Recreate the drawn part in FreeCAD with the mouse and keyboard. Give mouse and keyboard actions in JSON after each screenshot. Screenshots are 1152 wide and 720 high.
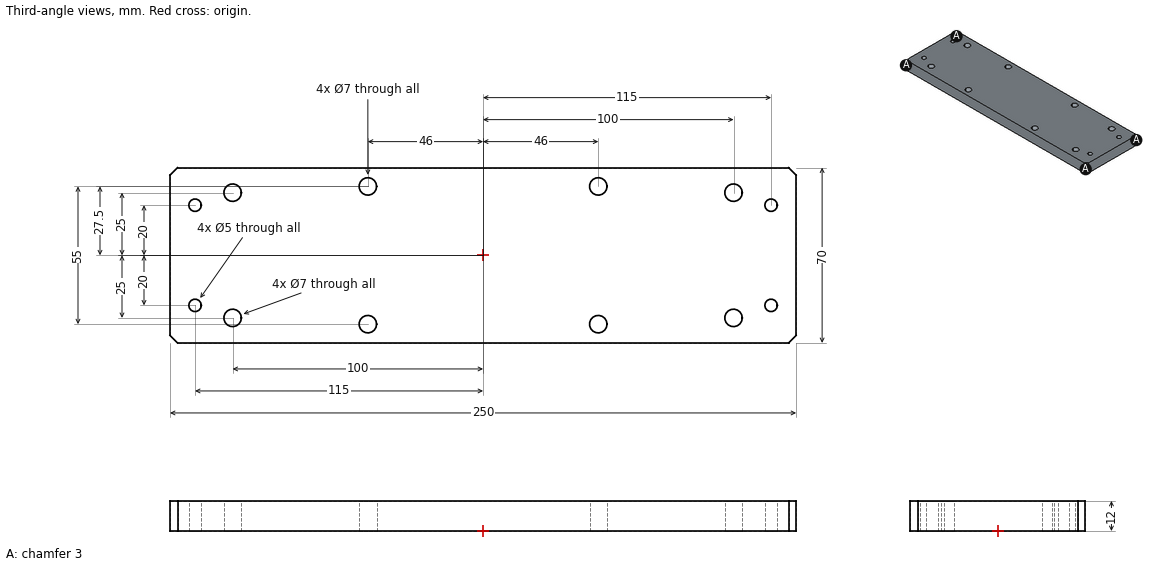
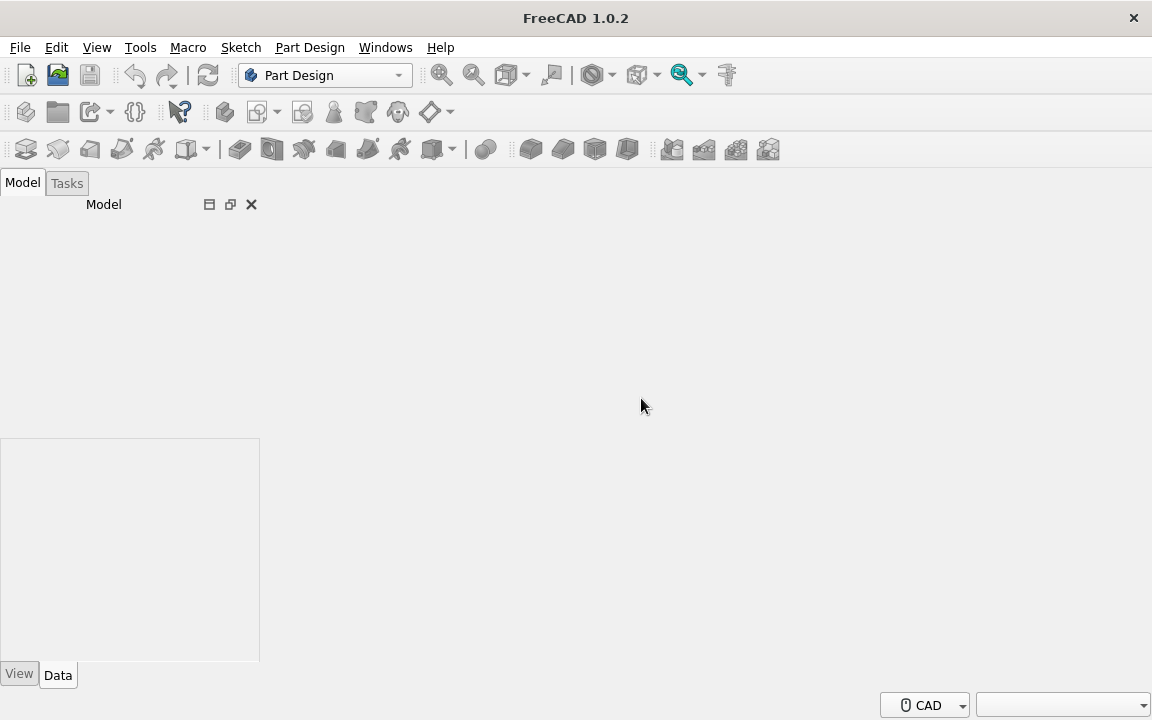
{"action": "key", "text": "ctrl+n"}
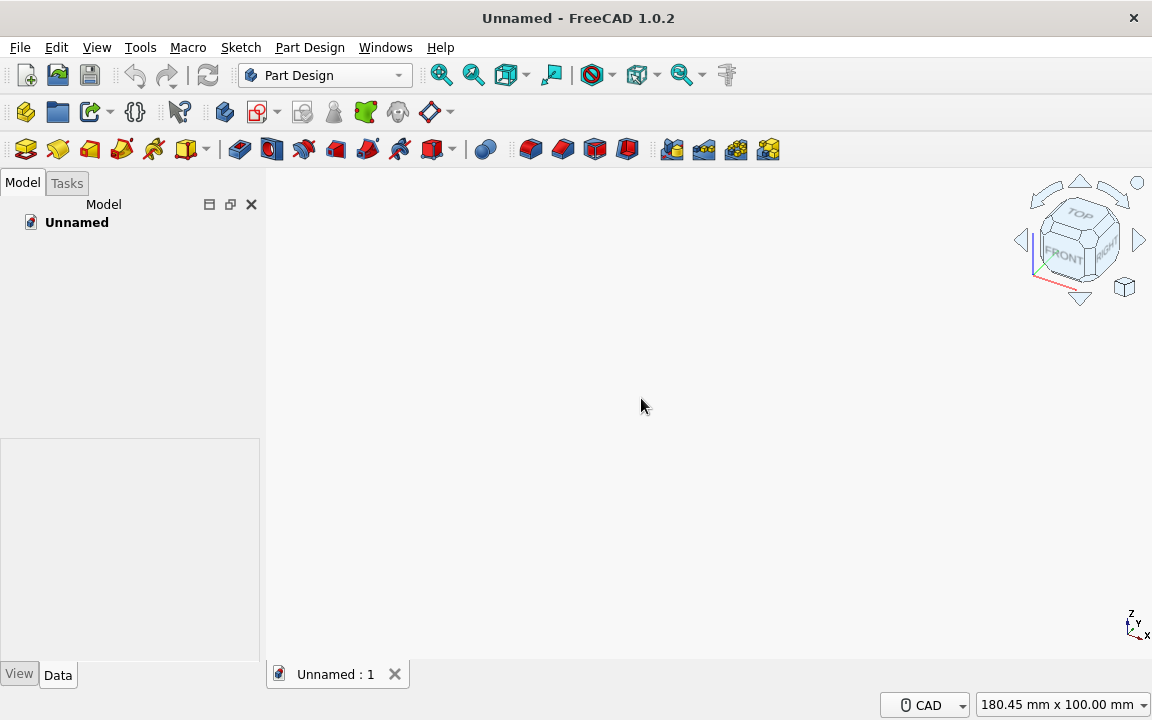
{"action": "left_click", "coordinate": [258, 112]}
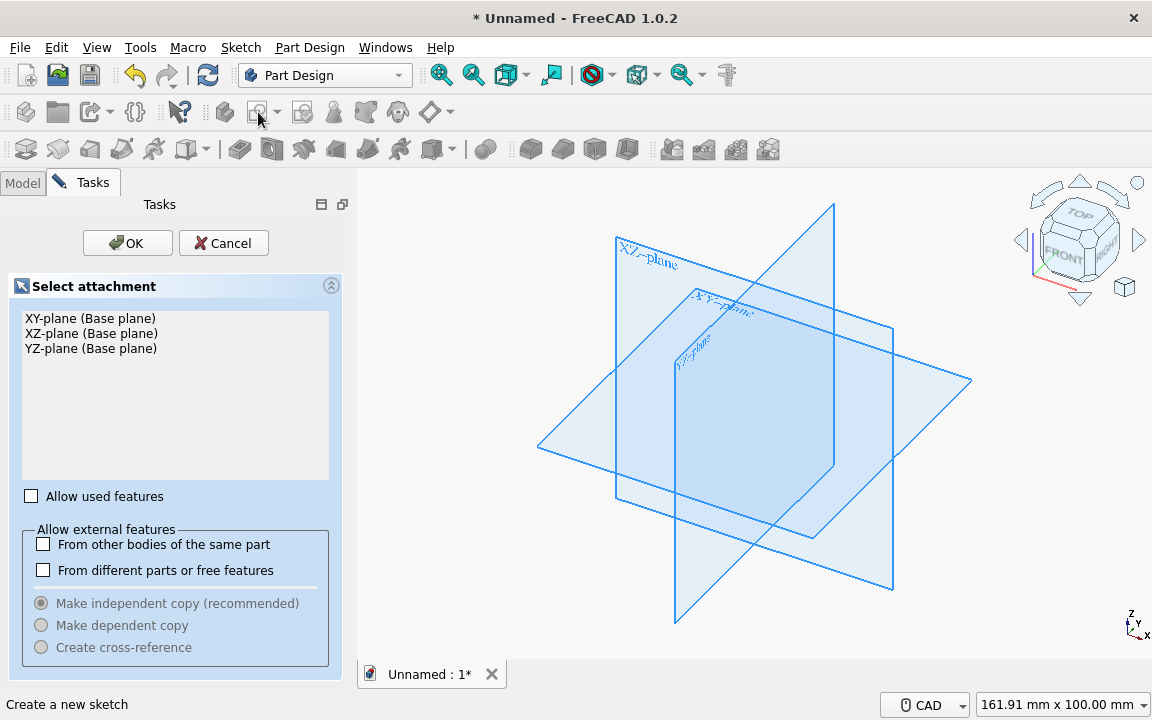
{"action": "left_click", "coordinate": [82, 318]}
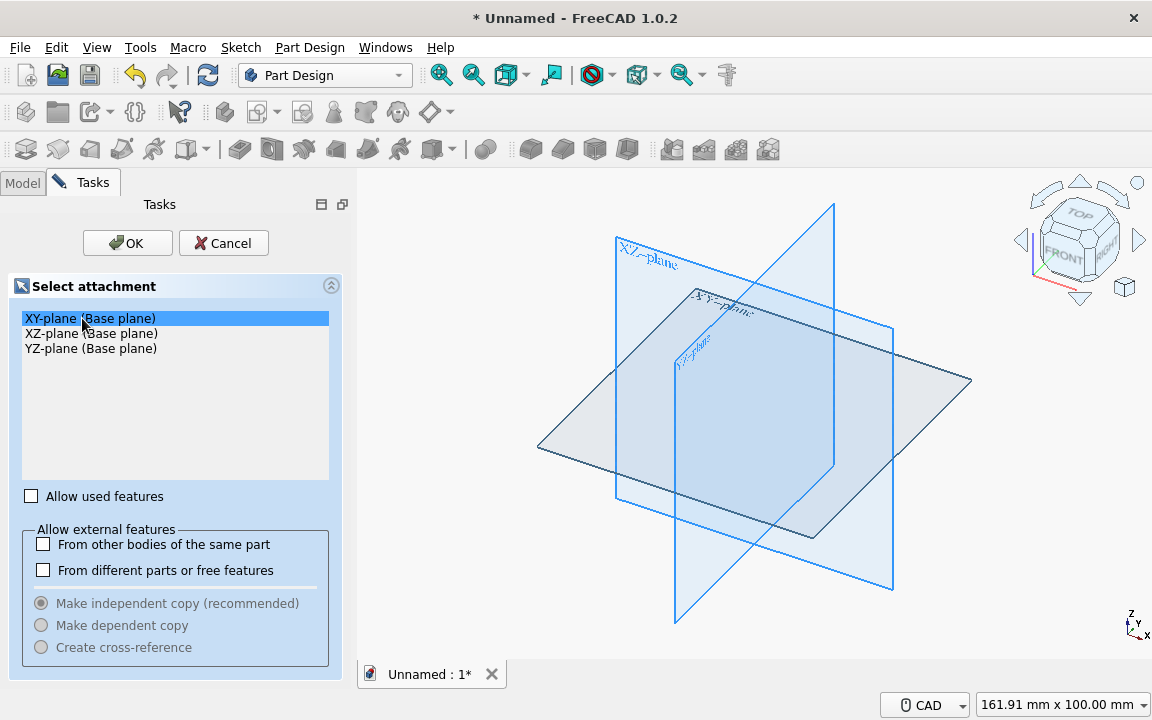
{"action": "left_click", "coordinate": [128, 243]}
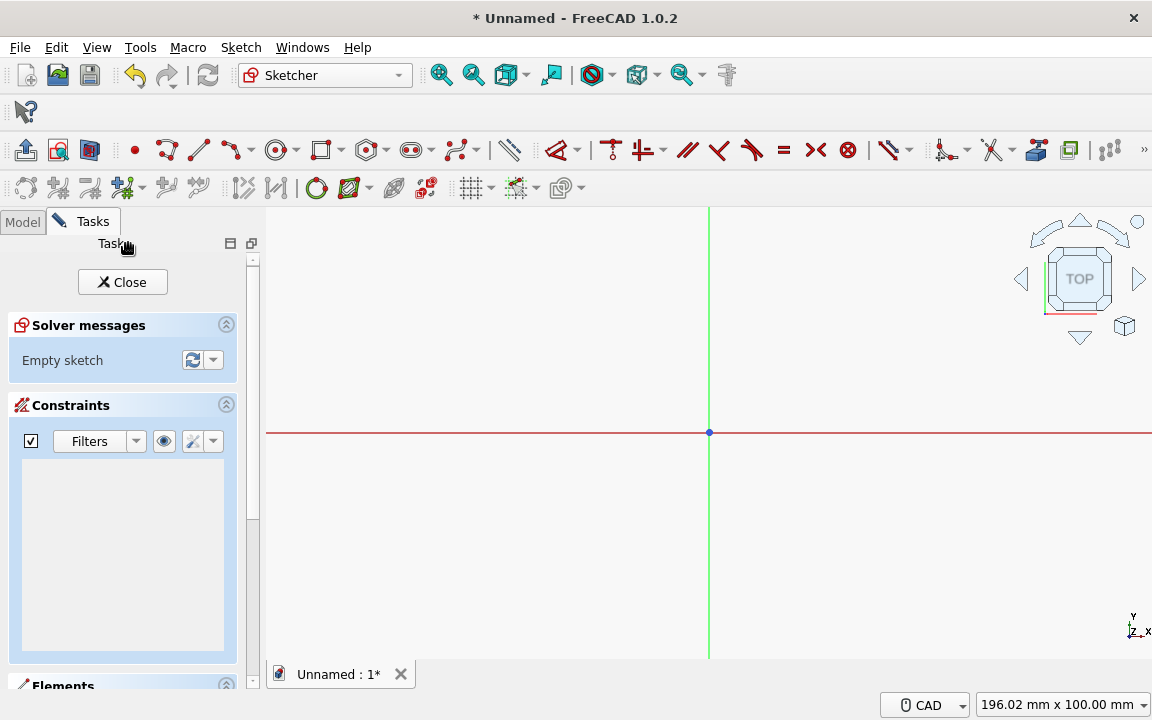
{"action": "scroll", "coordinate": [585, 433], "scroll_direction": "down", "scroll_amount": 4}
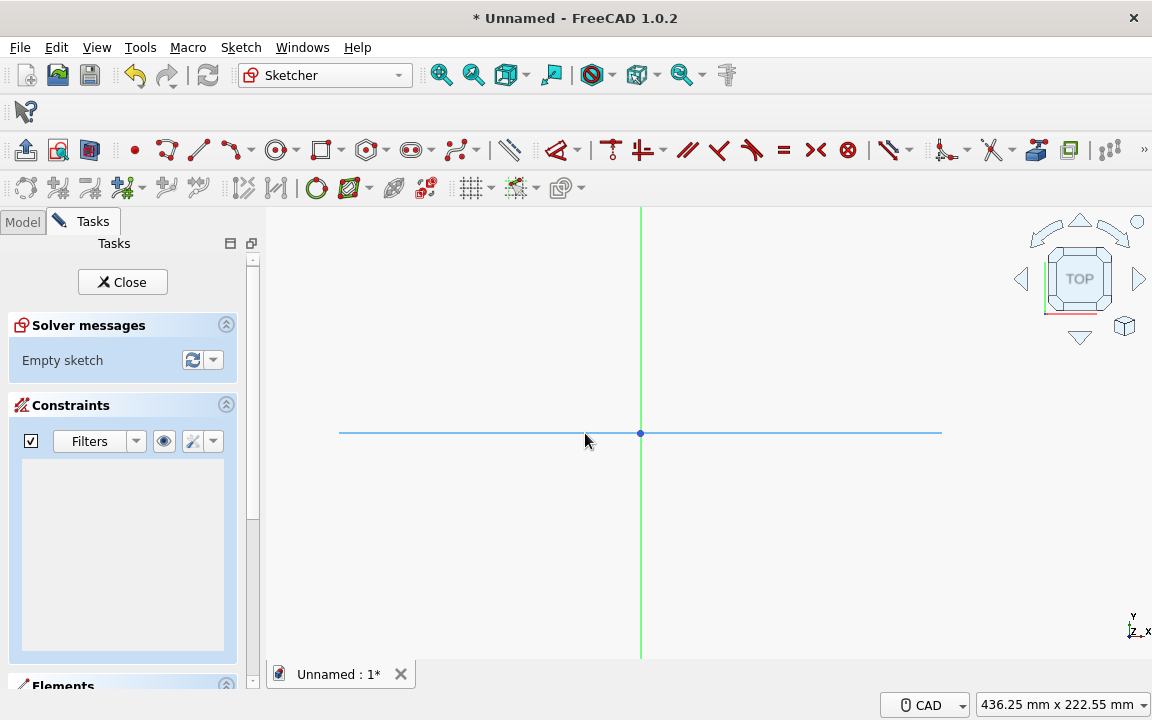
{"action": "left_click", "coordinate": [344, 150]}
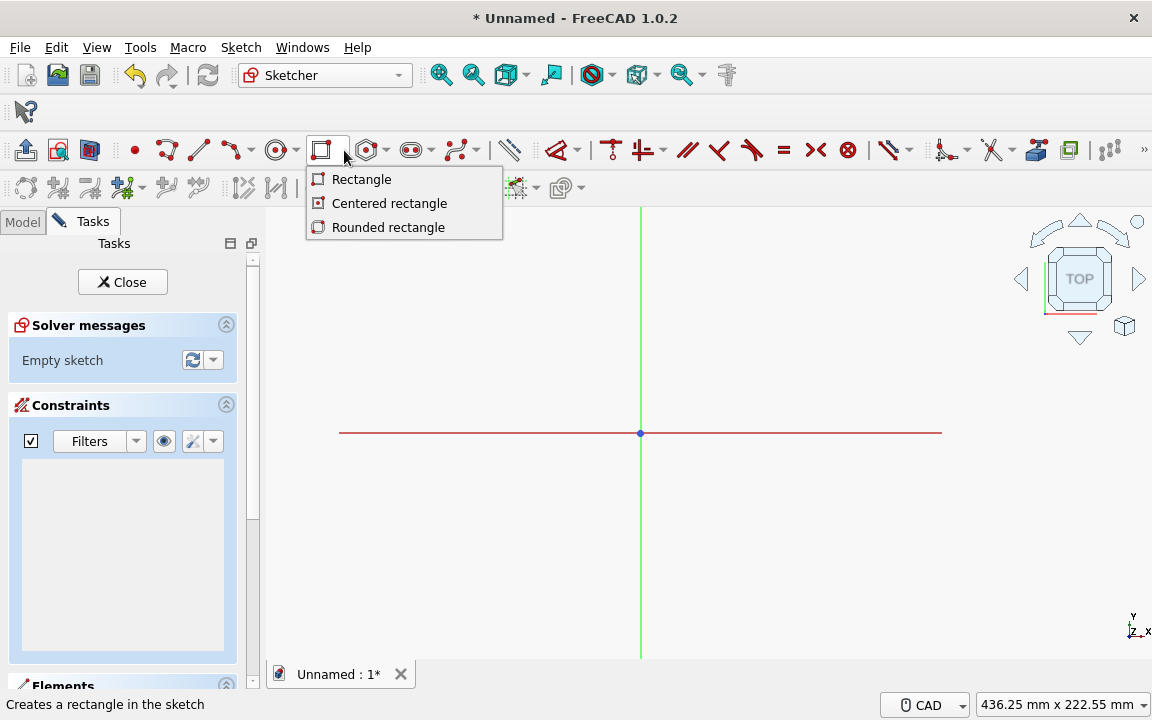
{"action": "left_click", "coordinate": [404, 203]}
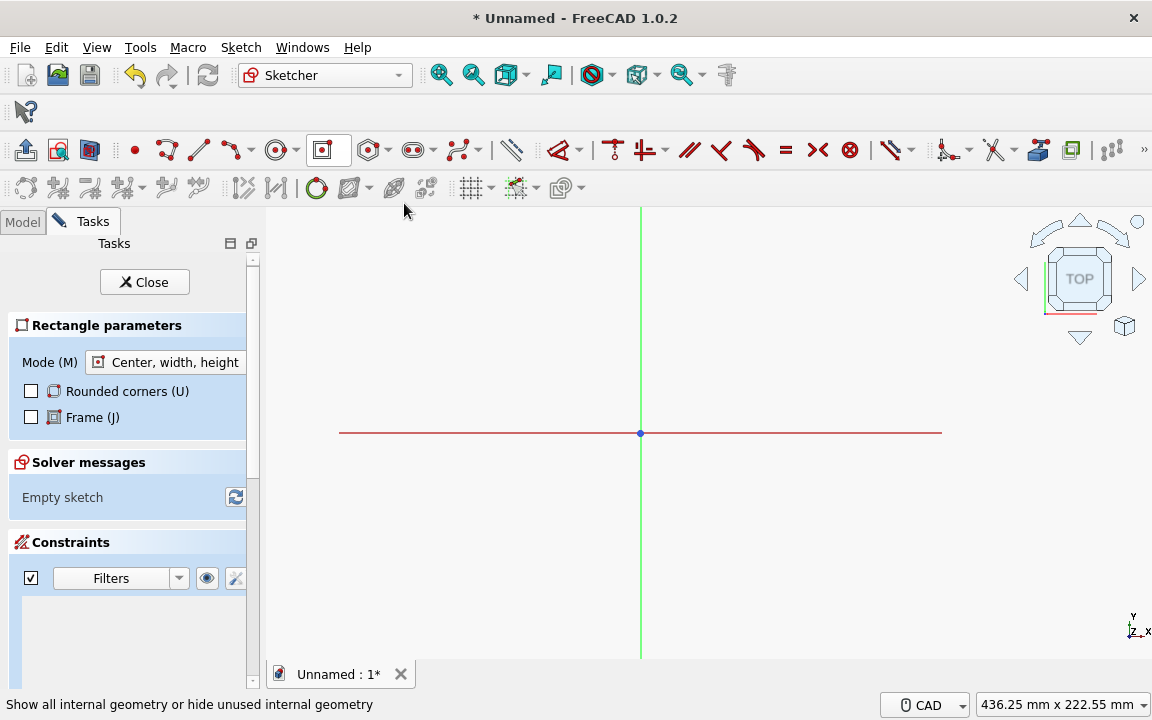
{"action": "left_click", "coordinate": [641, 433]}
{"action": "left_click", "coordinate": [895, 362]}
{"action": "key", "text": "Escape"}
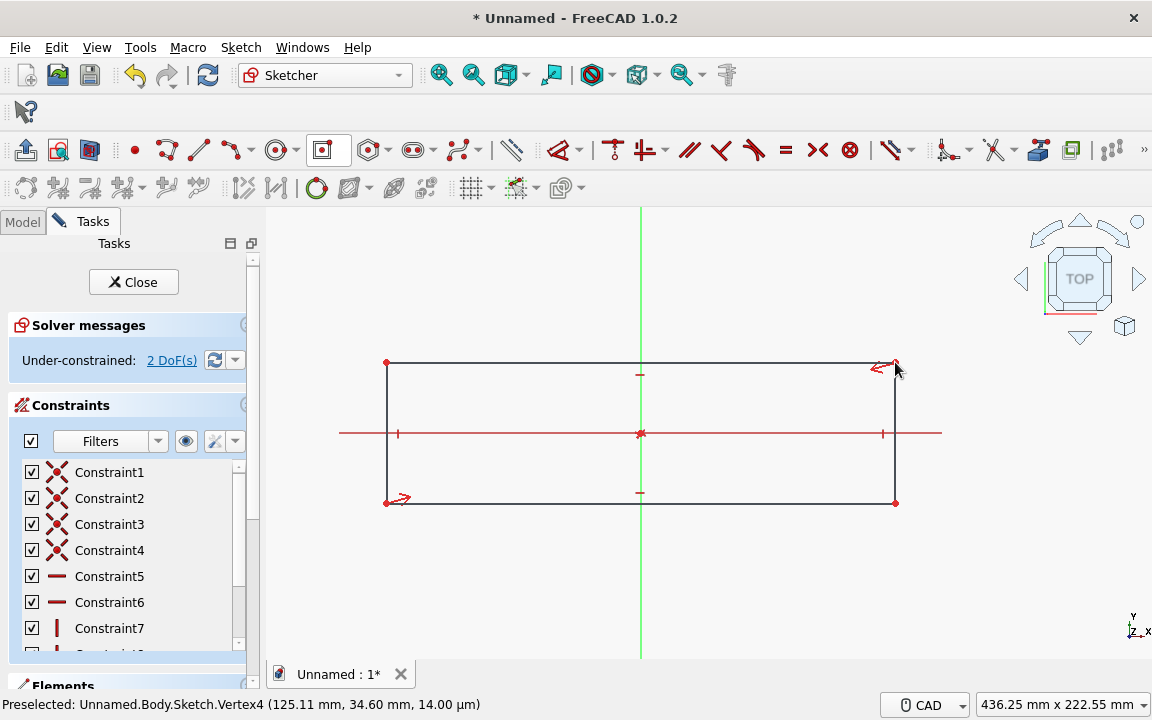
{"action": "left_click", "coordinate": [895, 461]}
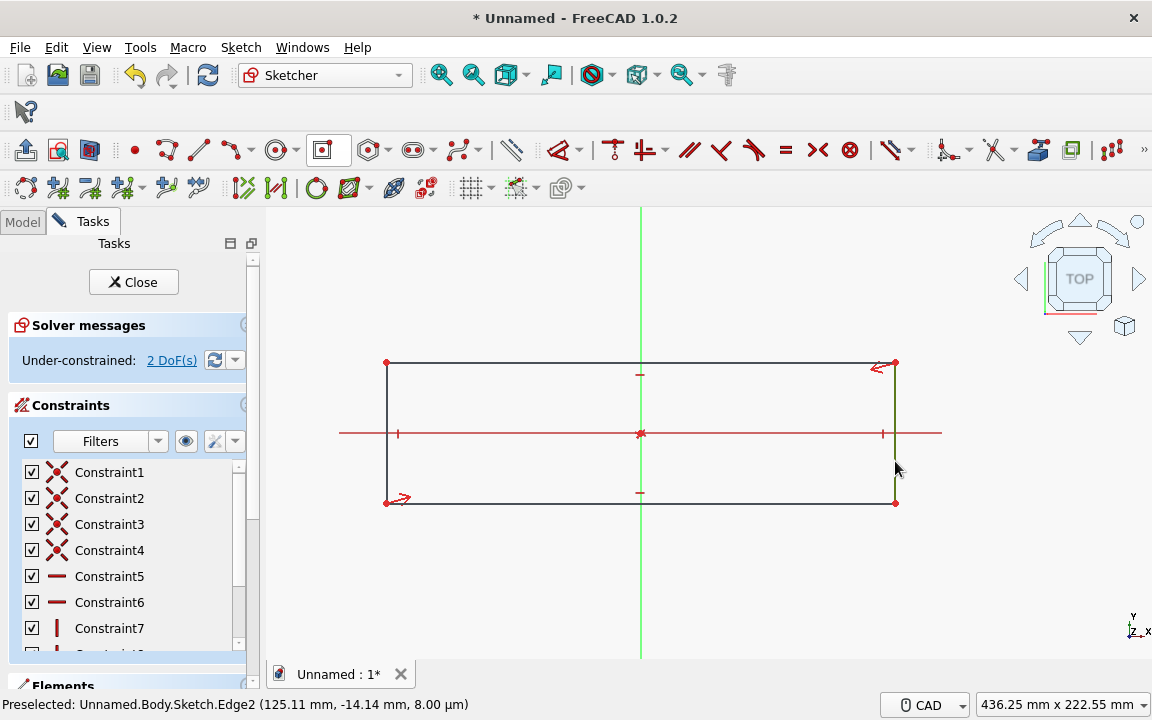
{"action": "key", "text": "i"}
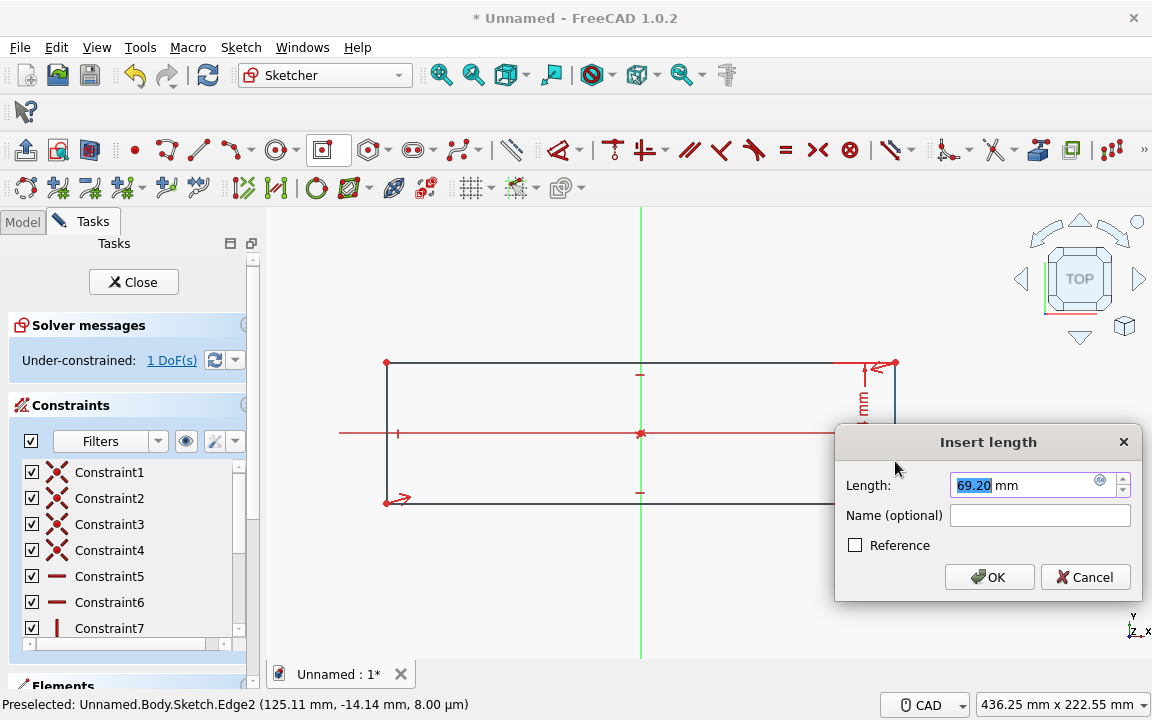
{"action": "type", "text": "70"}
{"action": "key", "text": "Return"}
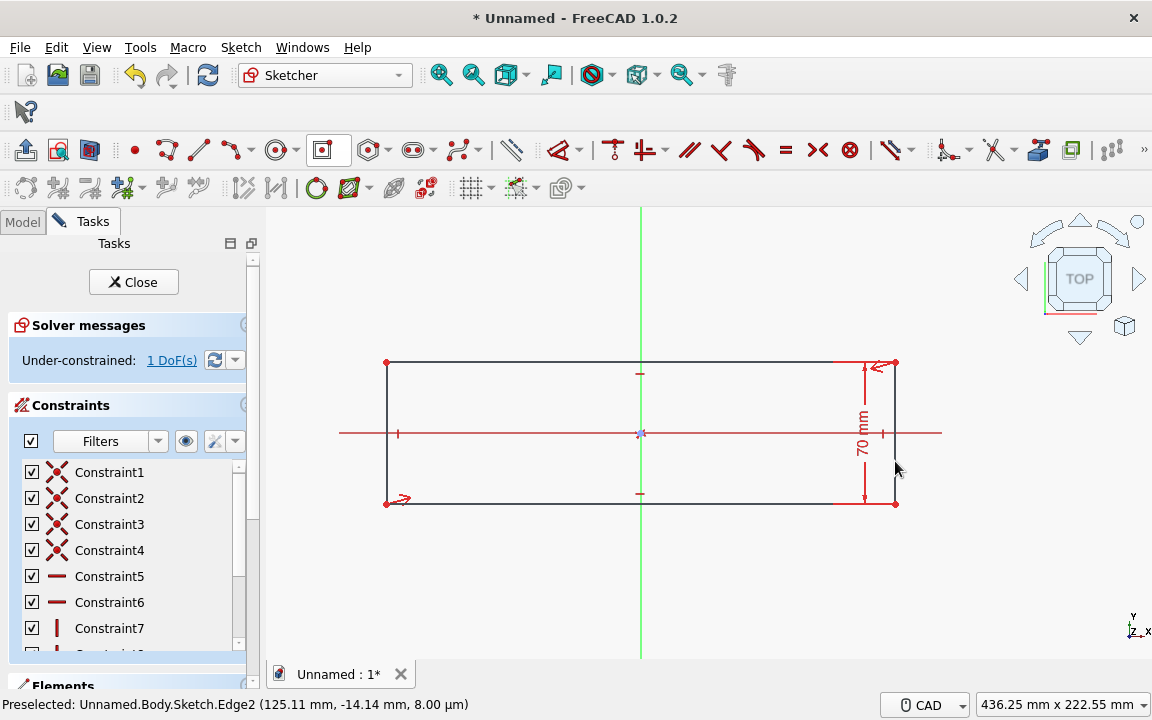
{"action": "left_click", "coordinate": [539, 504]}